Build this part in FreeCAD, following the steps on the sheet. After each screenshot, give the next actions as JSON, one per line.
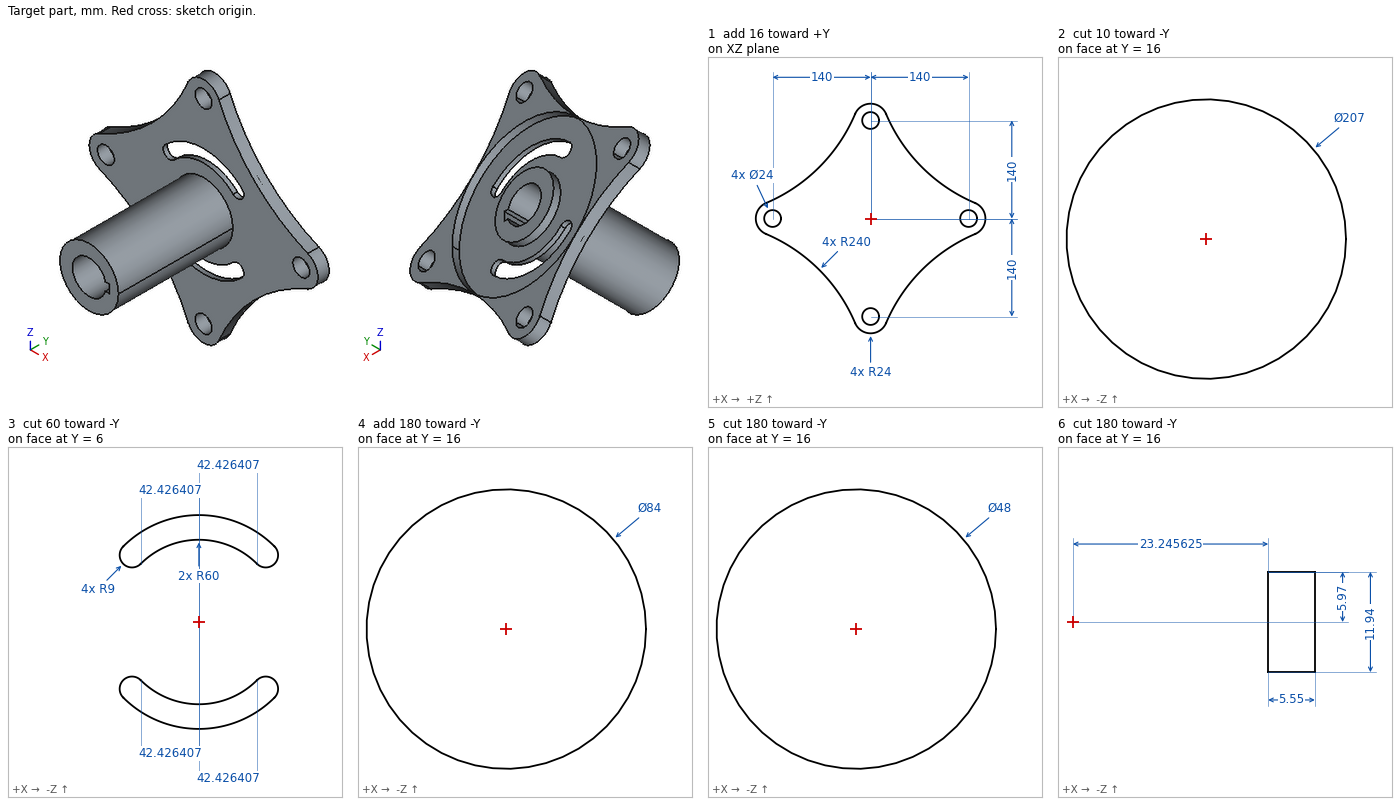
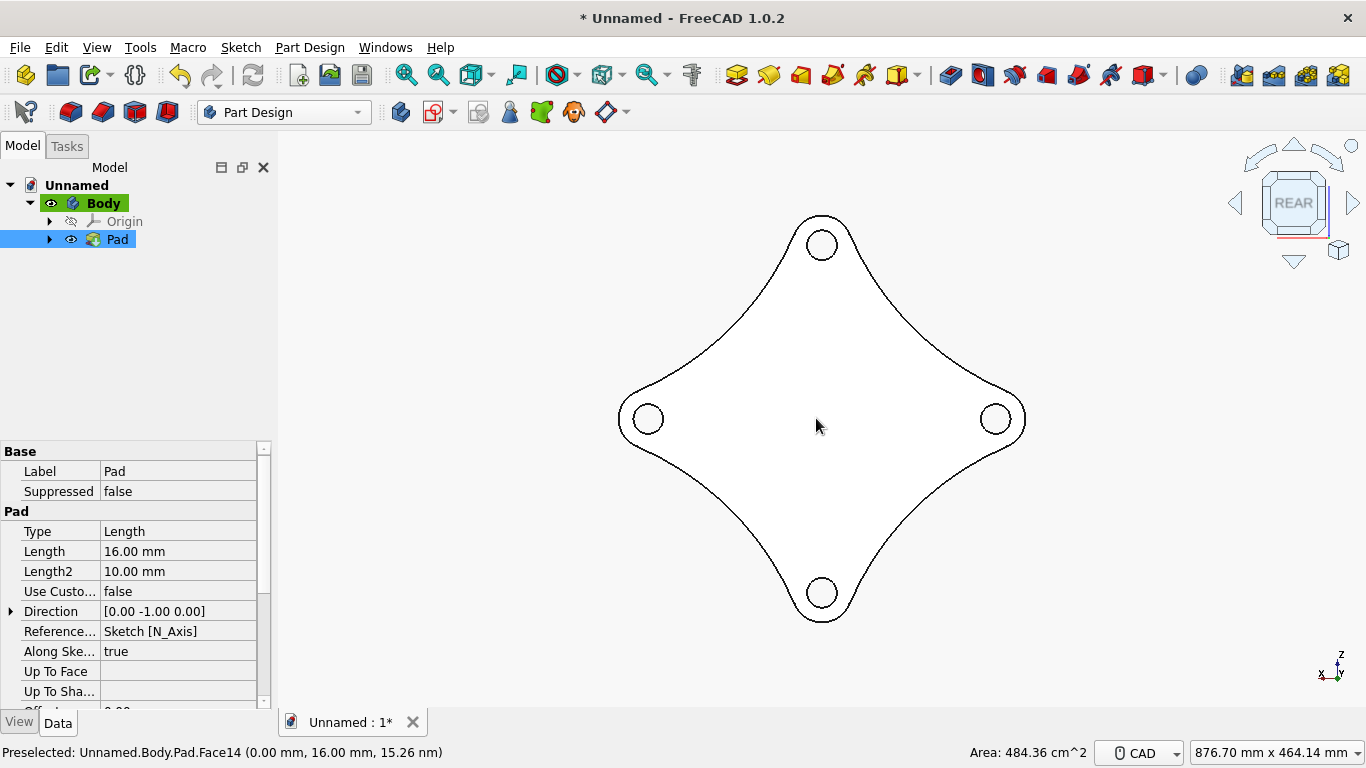
{"action": "left_click", "coordinate": [434, 112]}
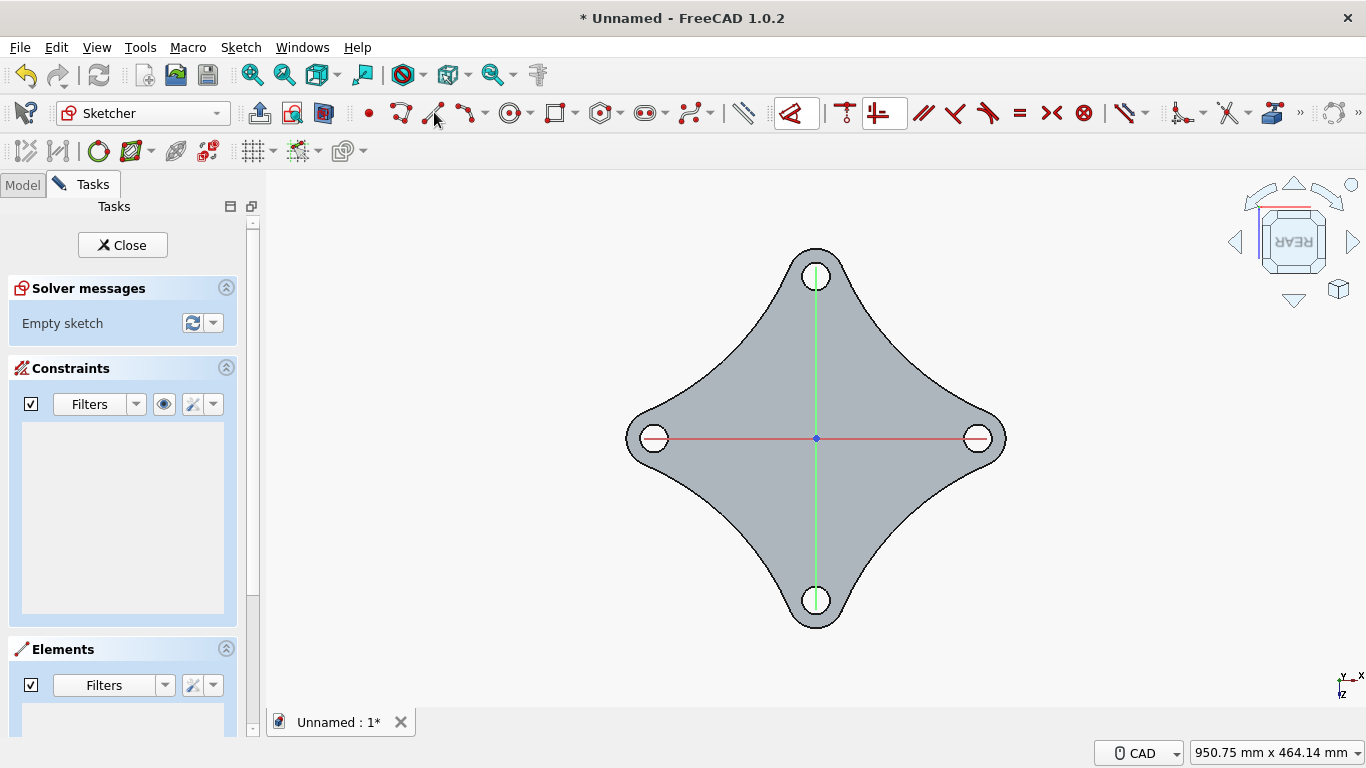
{"action": "scroll", "coordinate": [955, 438], "scroll_direction": "up", "scroll_amount": 2}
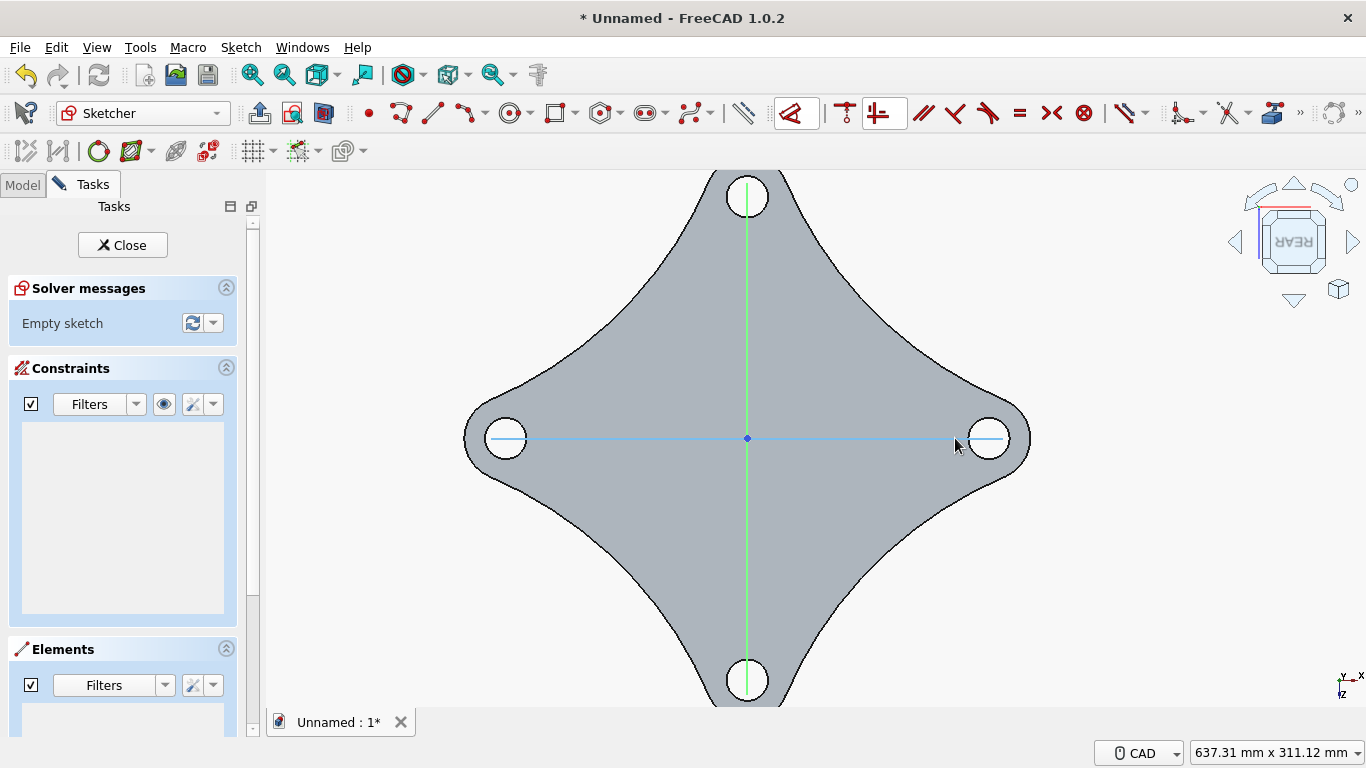
{"action": "left_click", "coordinate": [510, 114]}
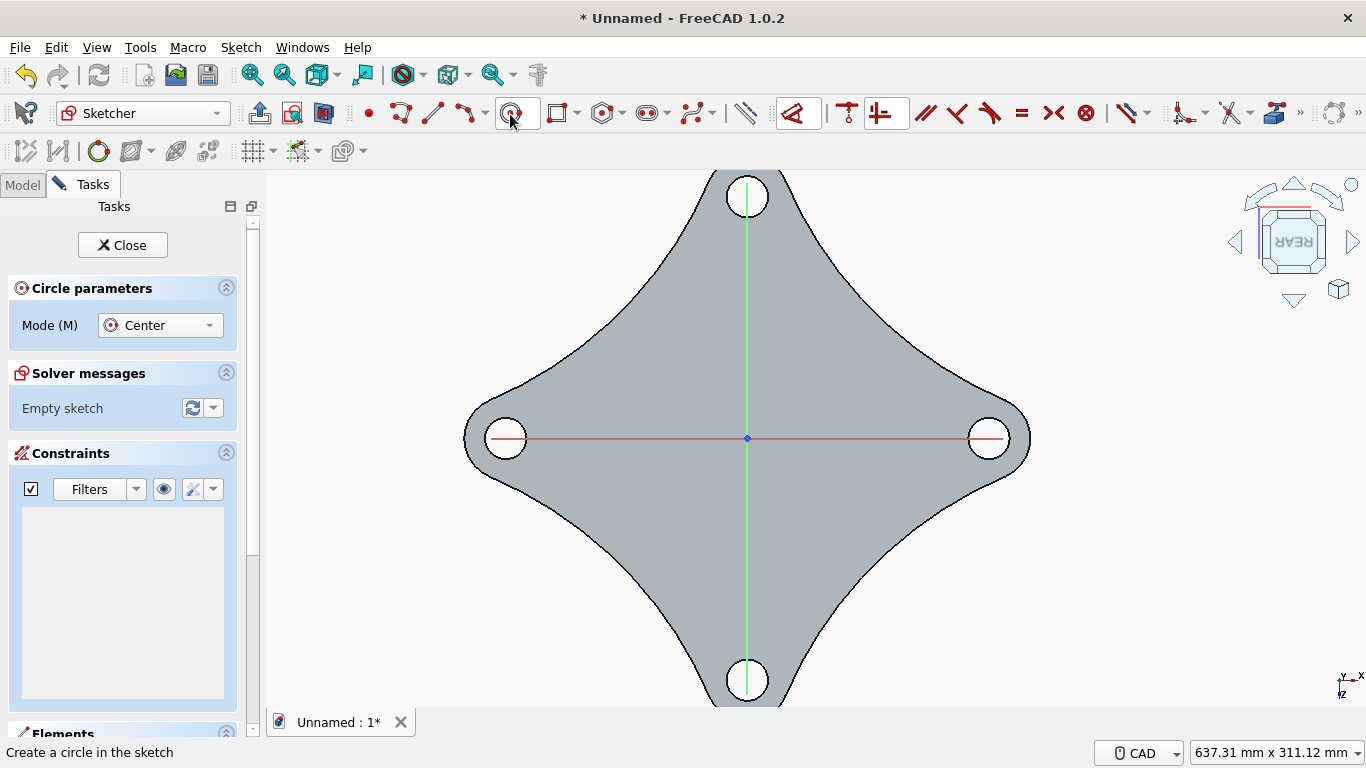
{"action": "left_click", "coordinate": [747, 438]}
{"action": "left_click", "coordinate": [874, 312]}
{"action": "key", "text": "Escape"}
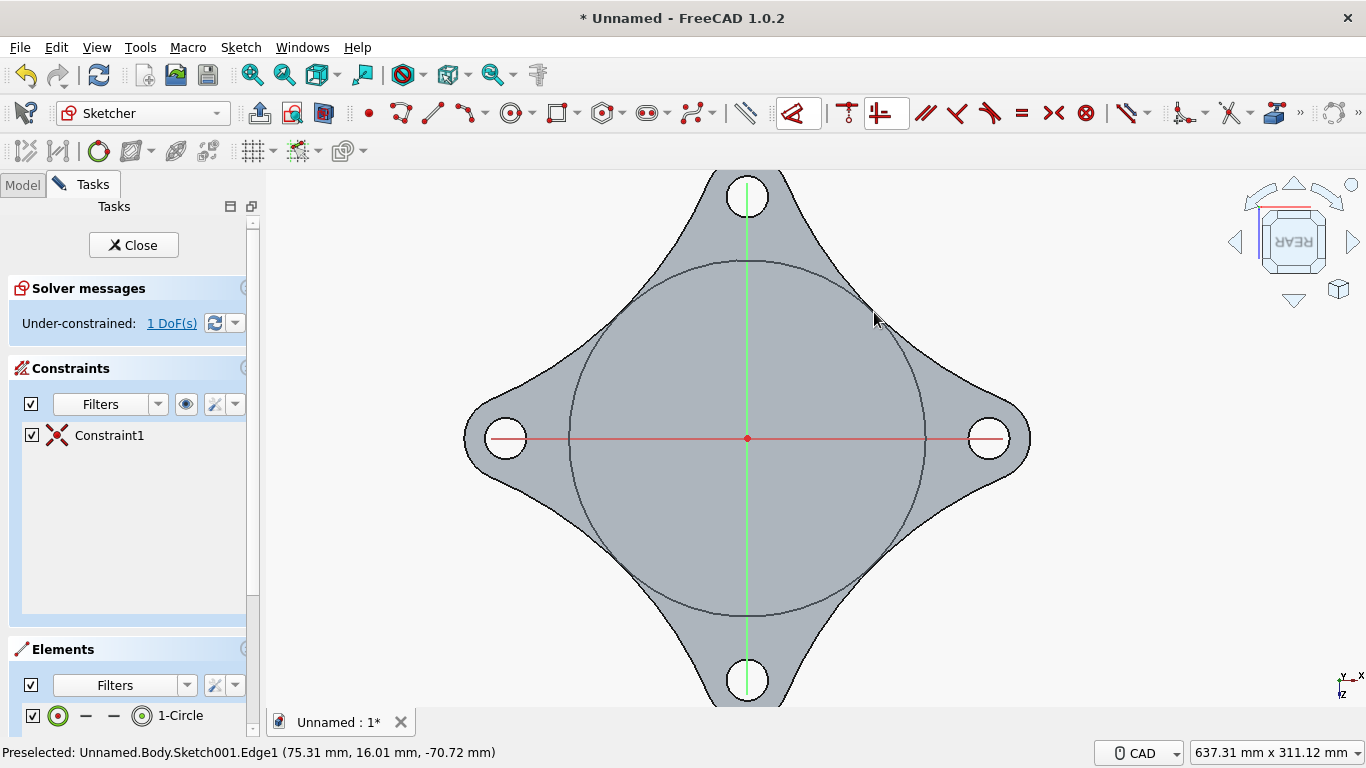
{"action": "left_click", "coordinate": [873, 312]}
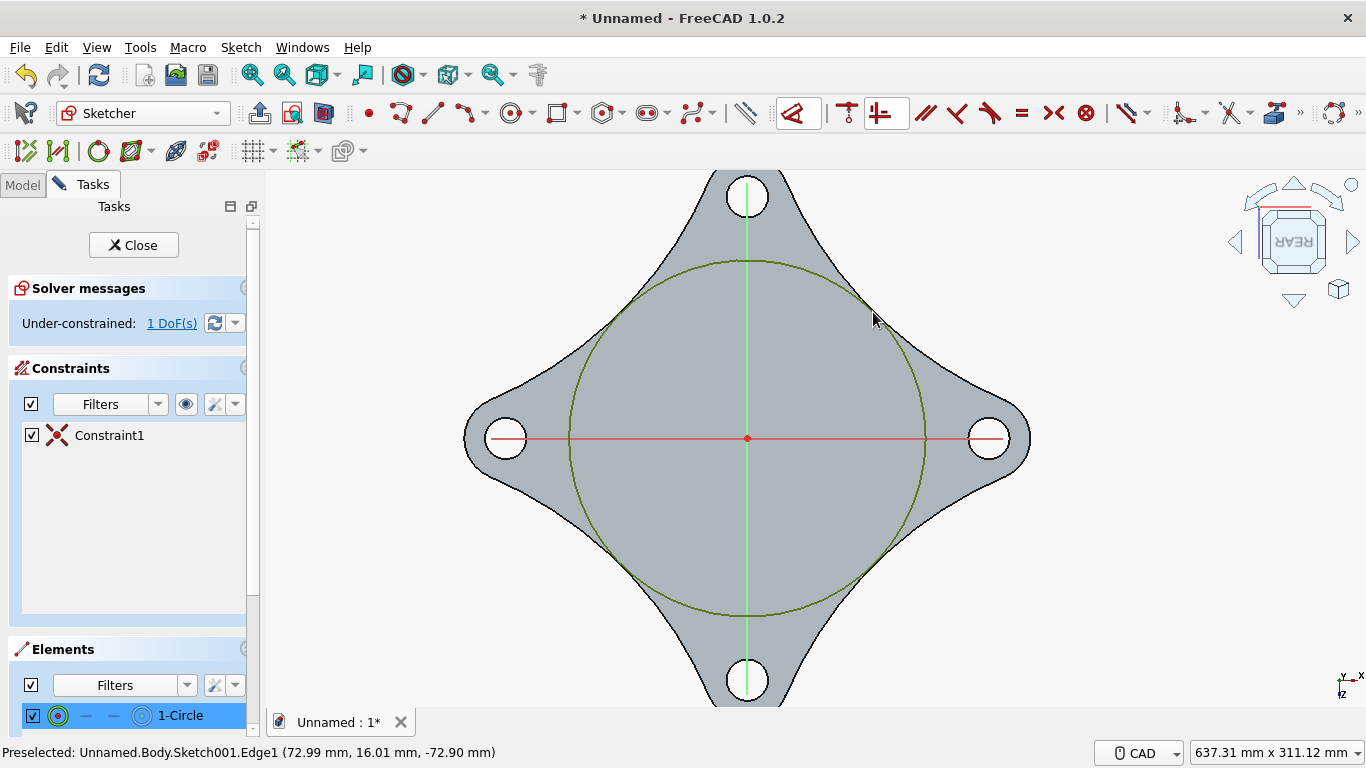
{"action": "key", "text": "k o"}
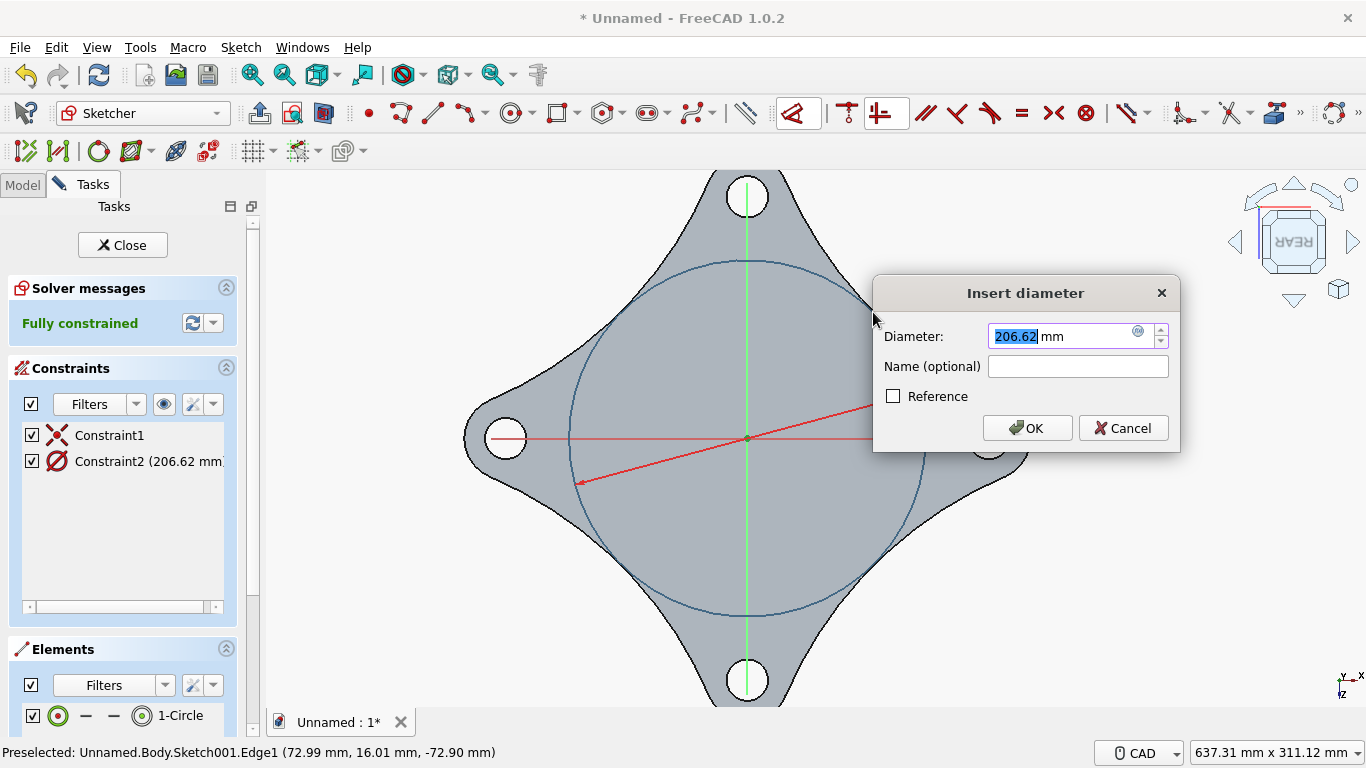
{"action": "type", "text": "207"}
{"action": "key", "text": "Return"}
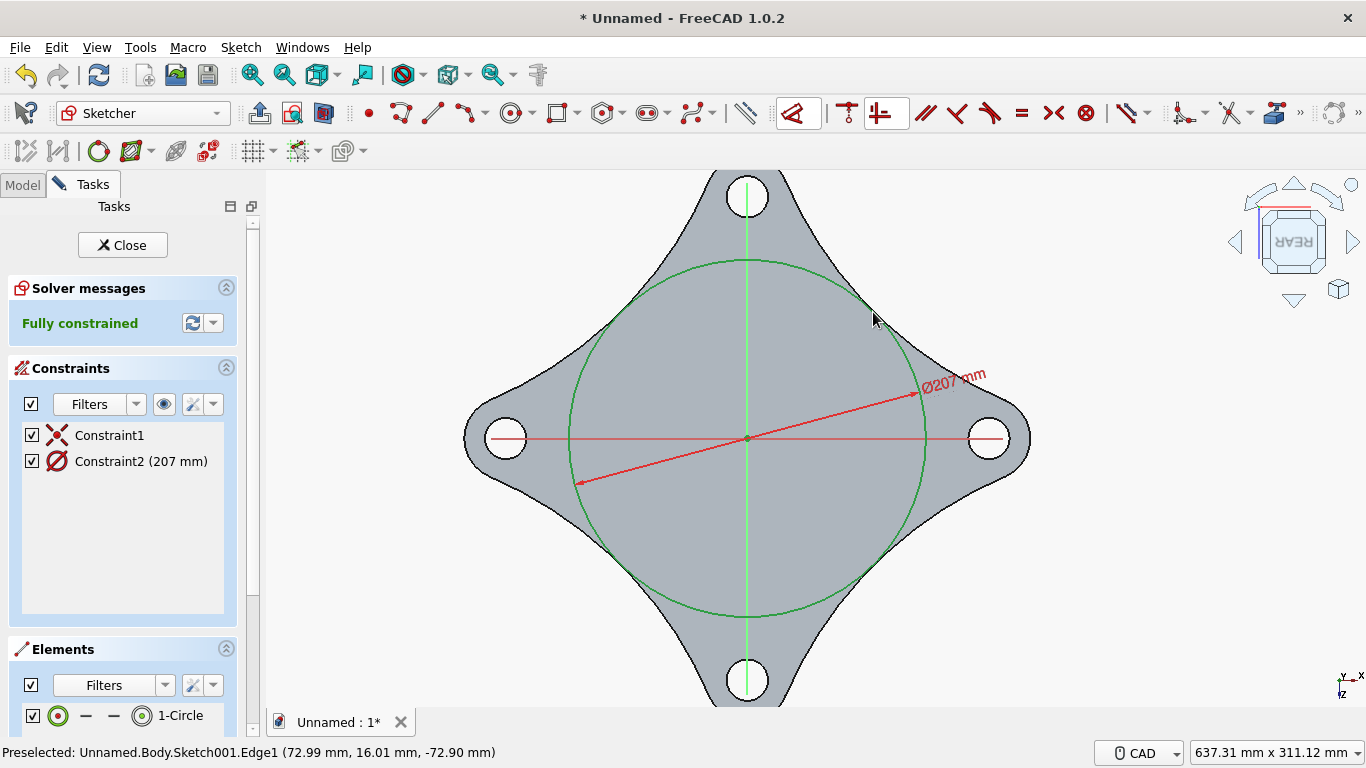
{"action": "left_click", "coordinate": [123, 245]}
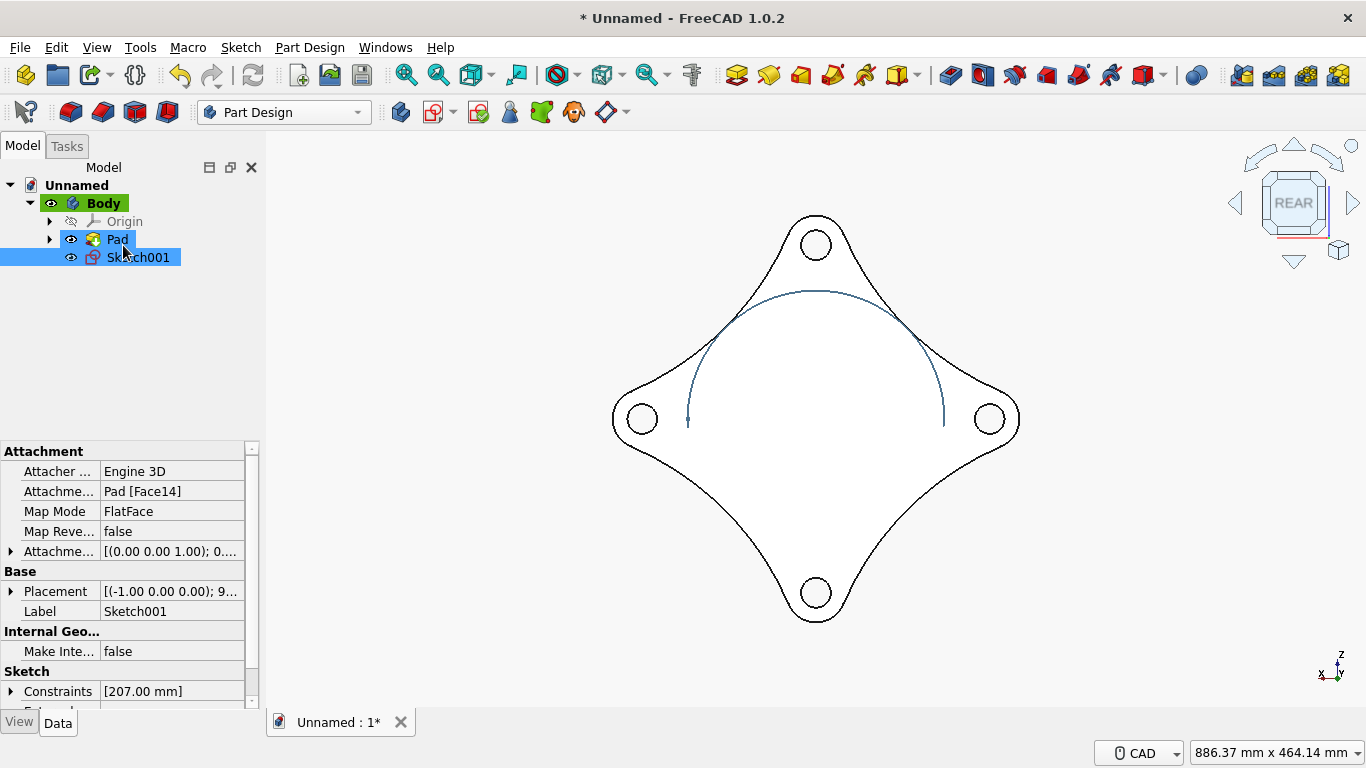
{"action": "left_click", "coordinate": [952, 76]}